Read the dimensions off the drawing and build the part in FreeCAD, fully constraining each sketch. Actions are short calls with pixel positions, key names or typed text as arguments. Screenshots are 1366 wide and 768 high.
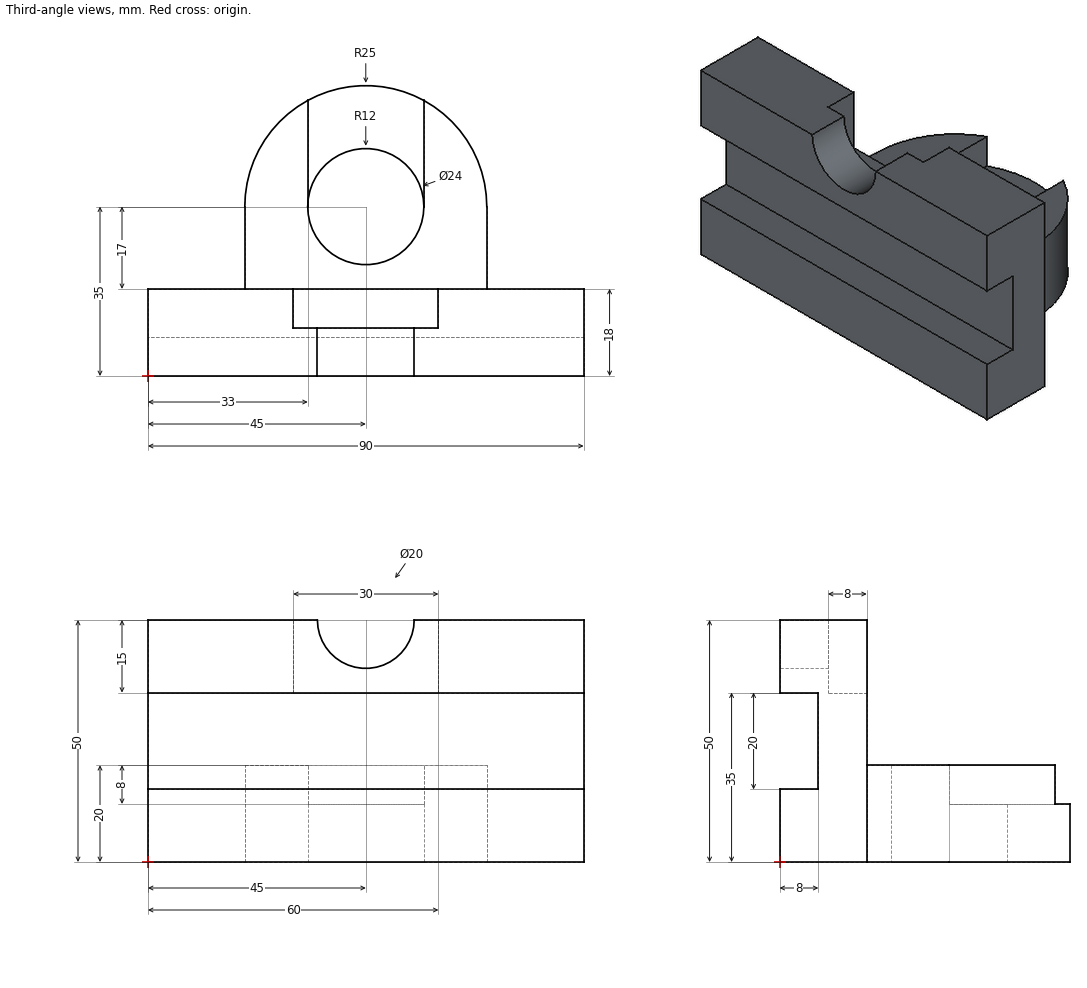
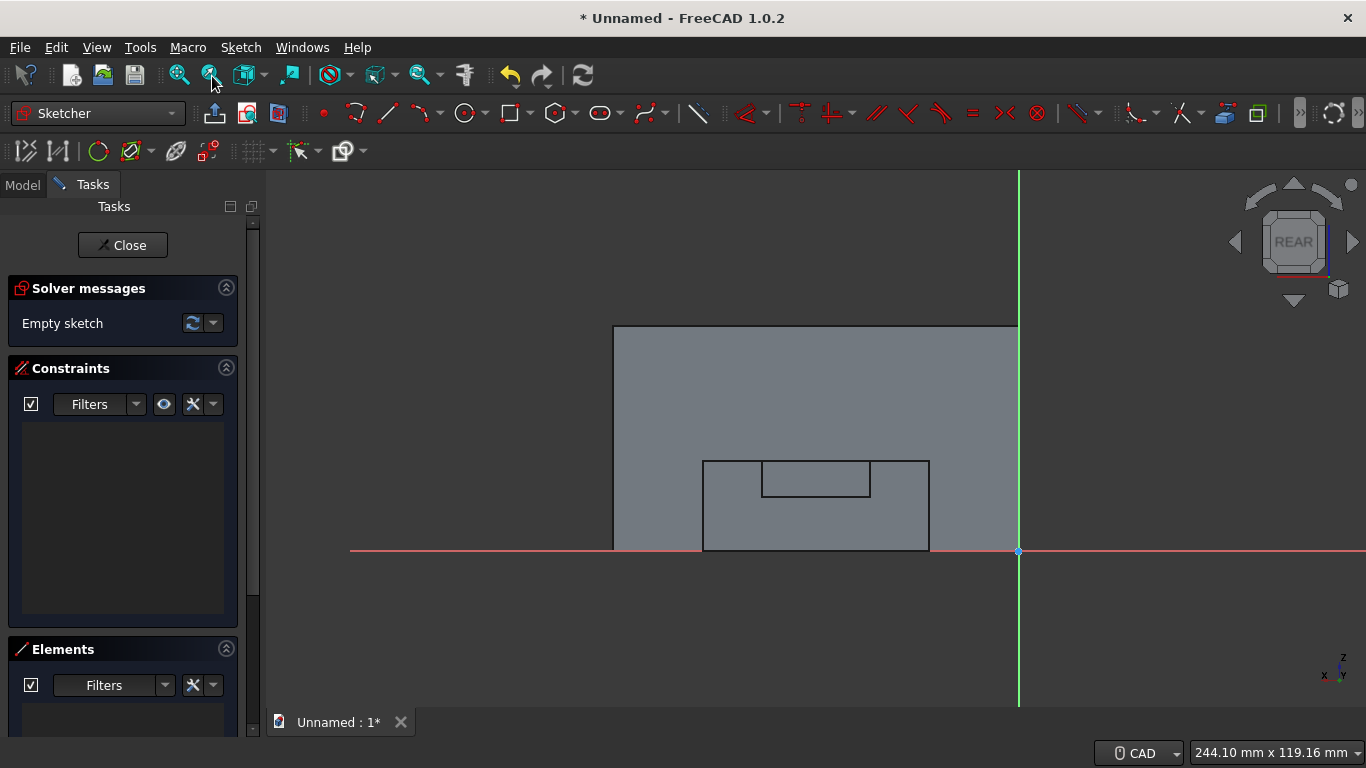
key(q)
key(s)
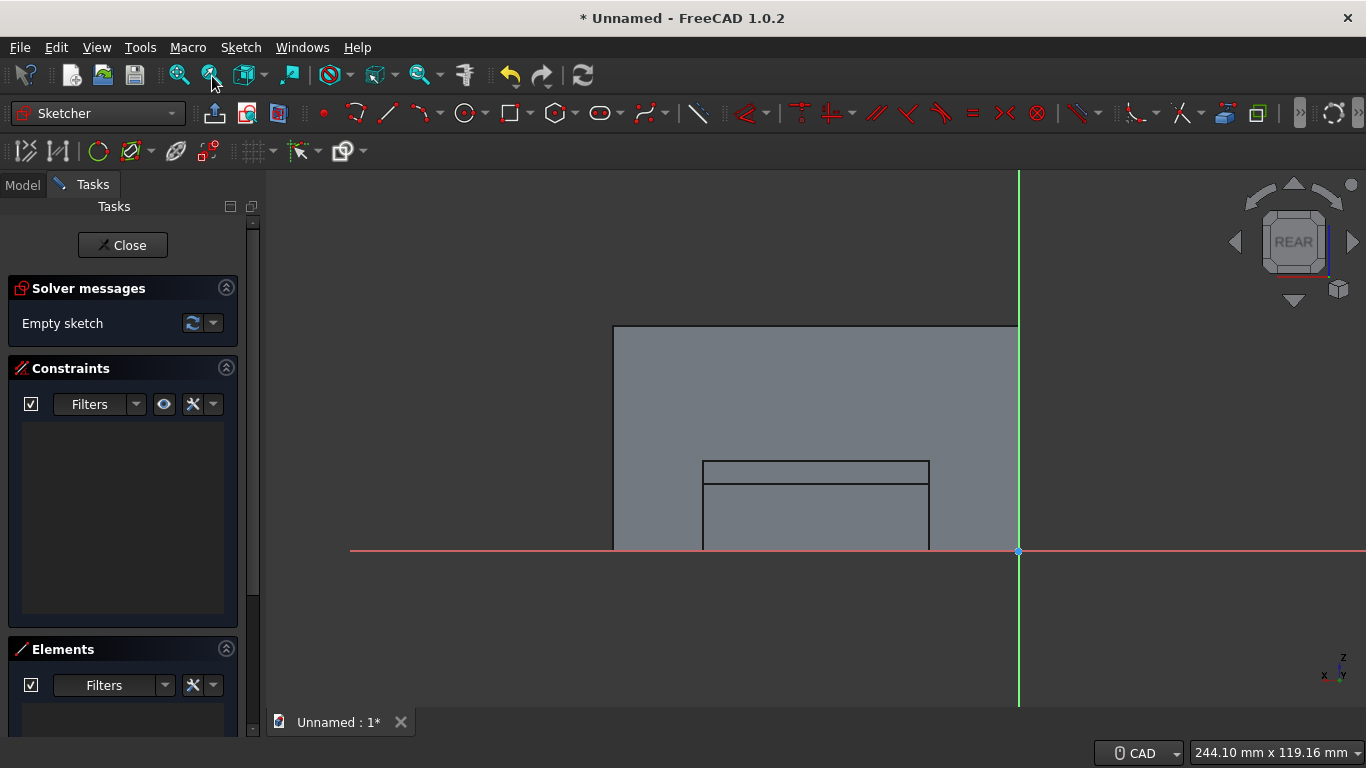
scroll(1160, 438, up, 2)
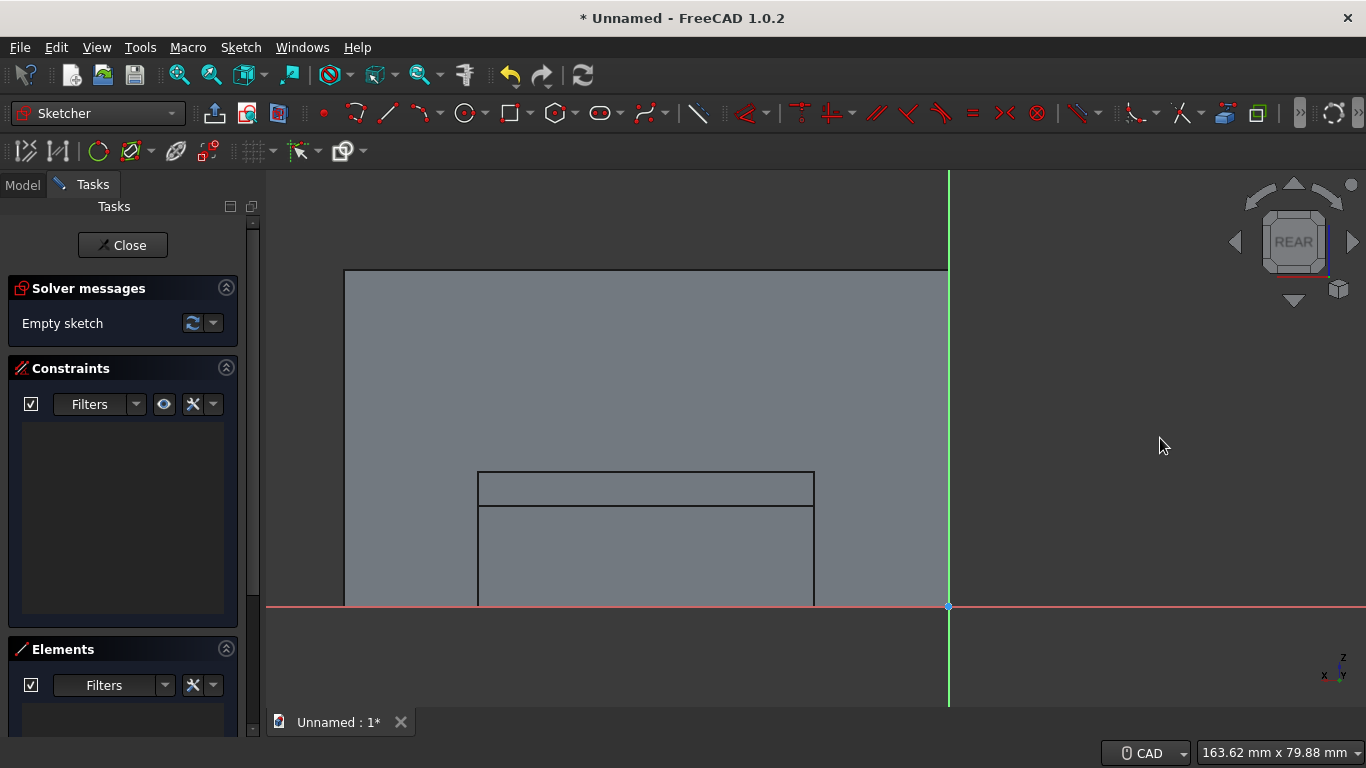
click(510, 114)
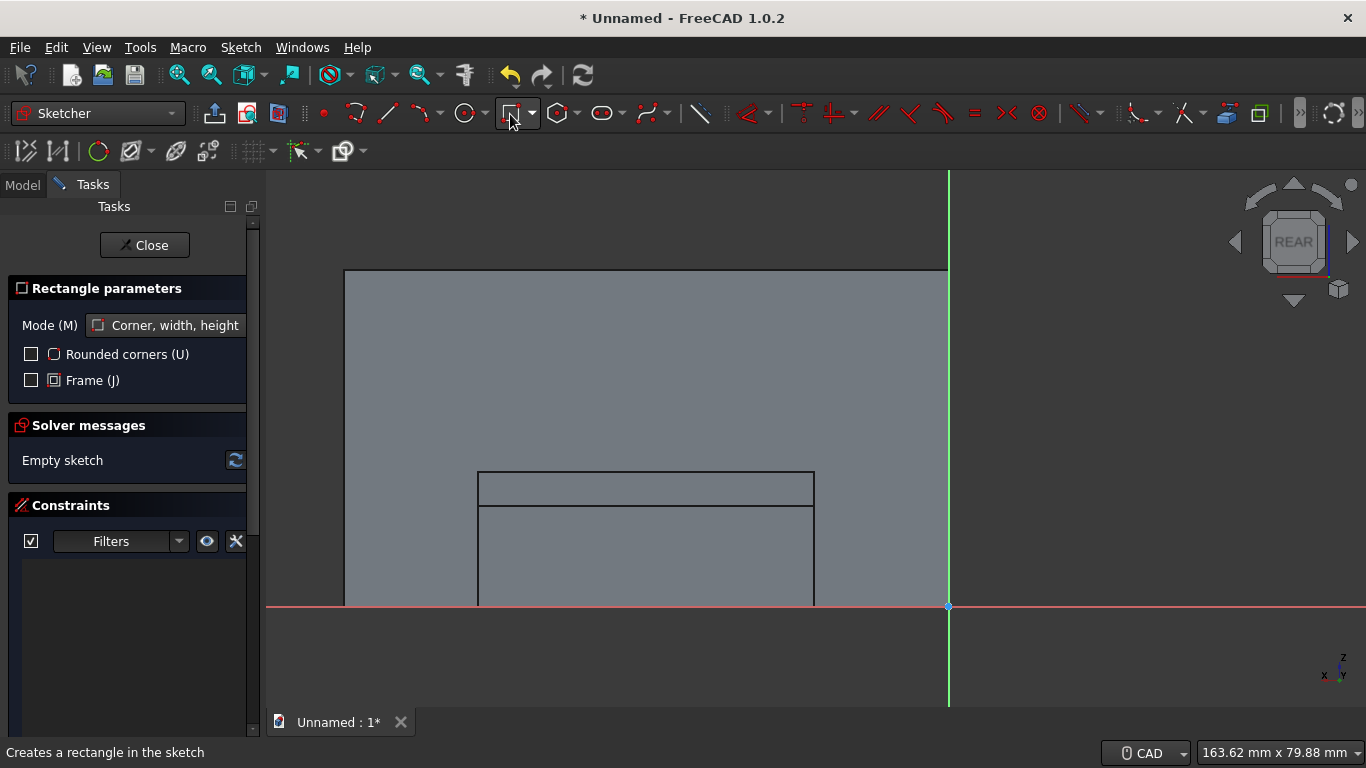
click(546, 270)
move(747, 371)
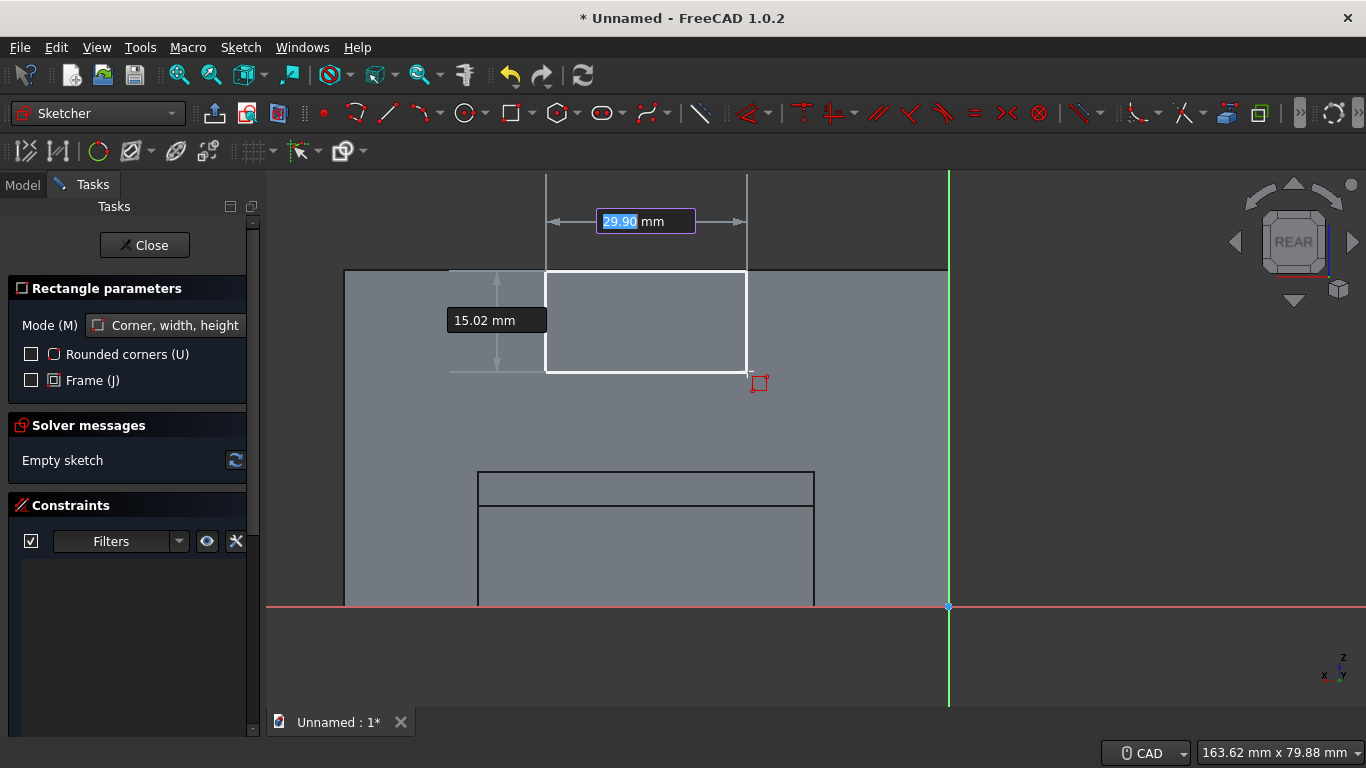
text(30)
key(Tab)
text(15)
key(Return)
key(Escape)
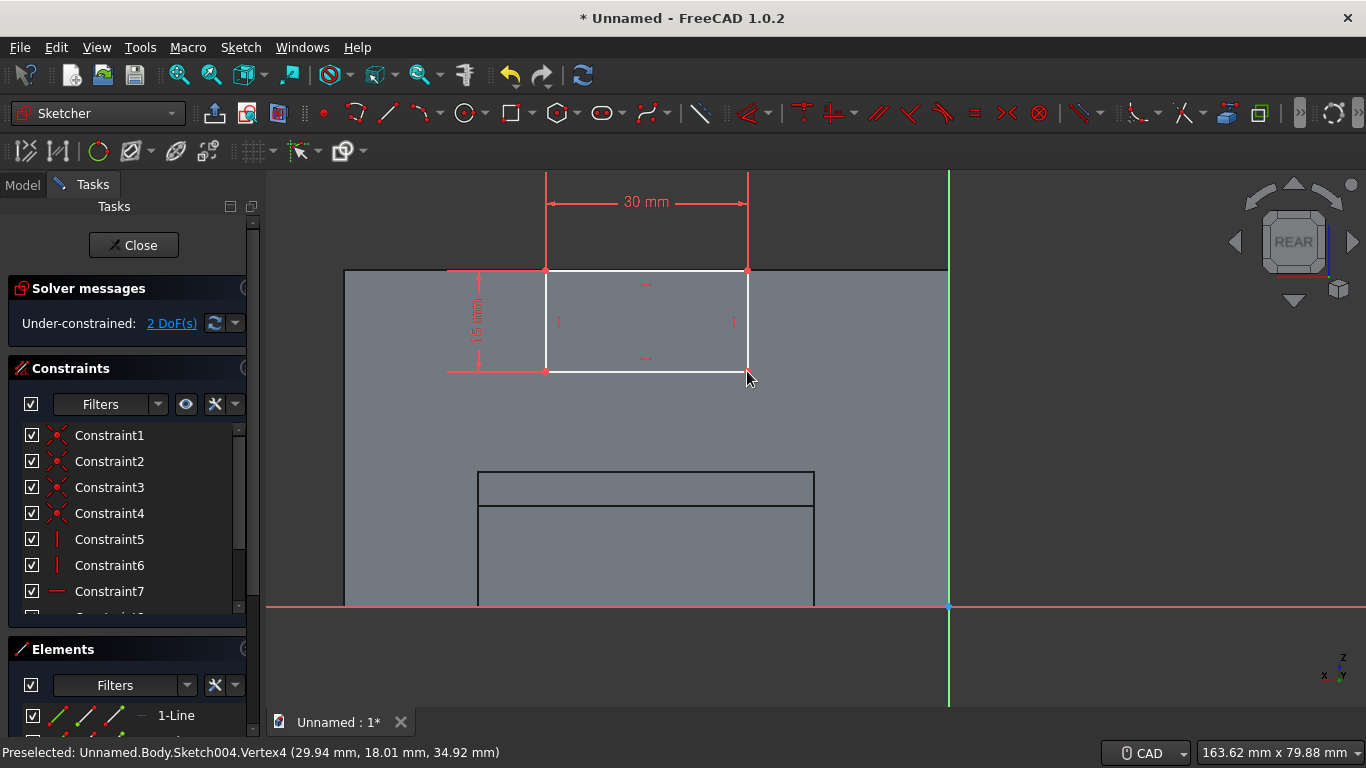
key(d)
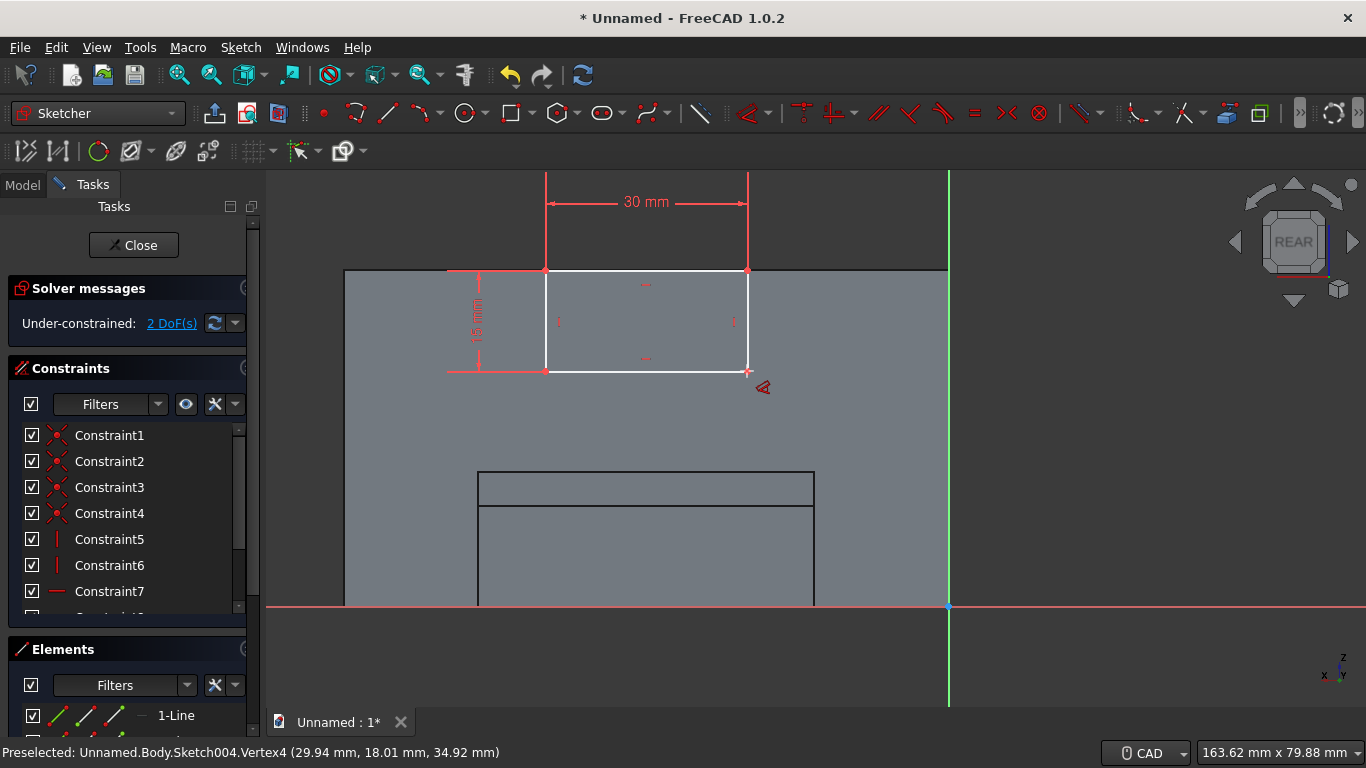
click(546, 271)
click(747, 641)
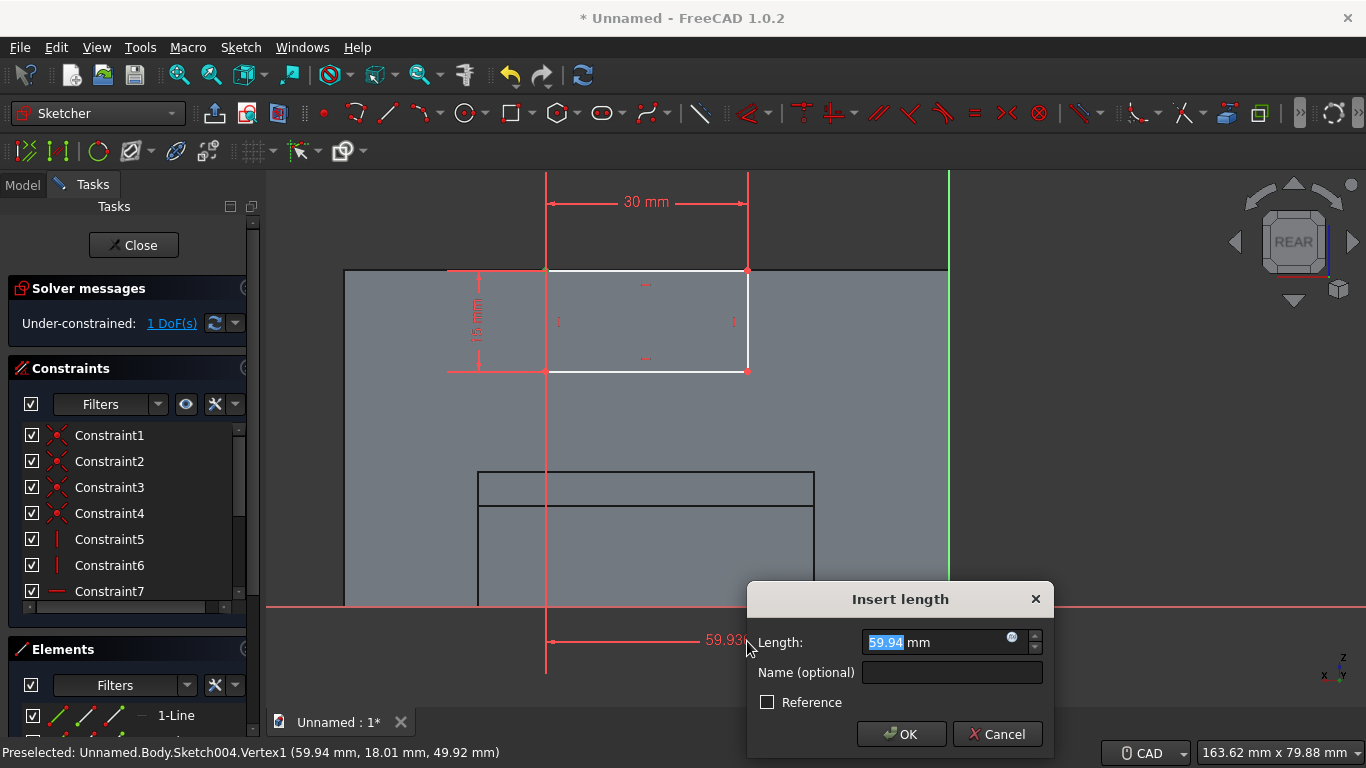
text(60)
key(Return)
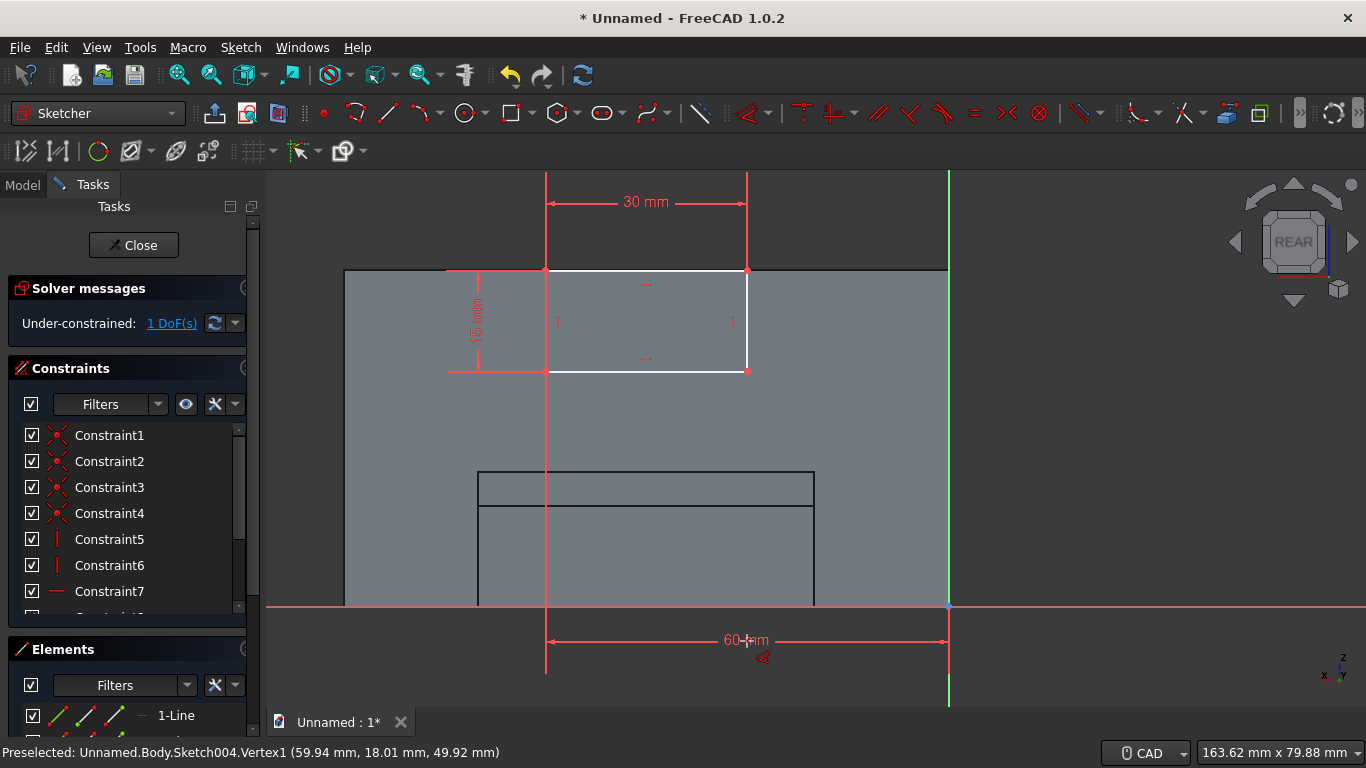
click(546, 271)
click(983, 439)